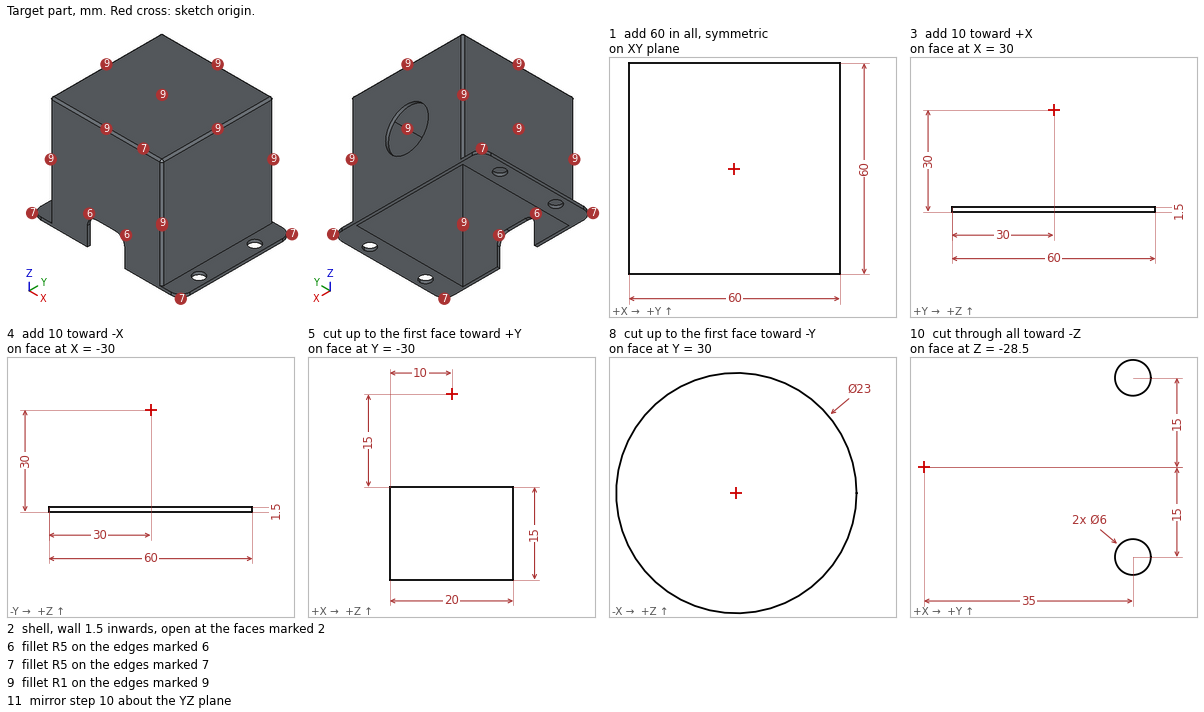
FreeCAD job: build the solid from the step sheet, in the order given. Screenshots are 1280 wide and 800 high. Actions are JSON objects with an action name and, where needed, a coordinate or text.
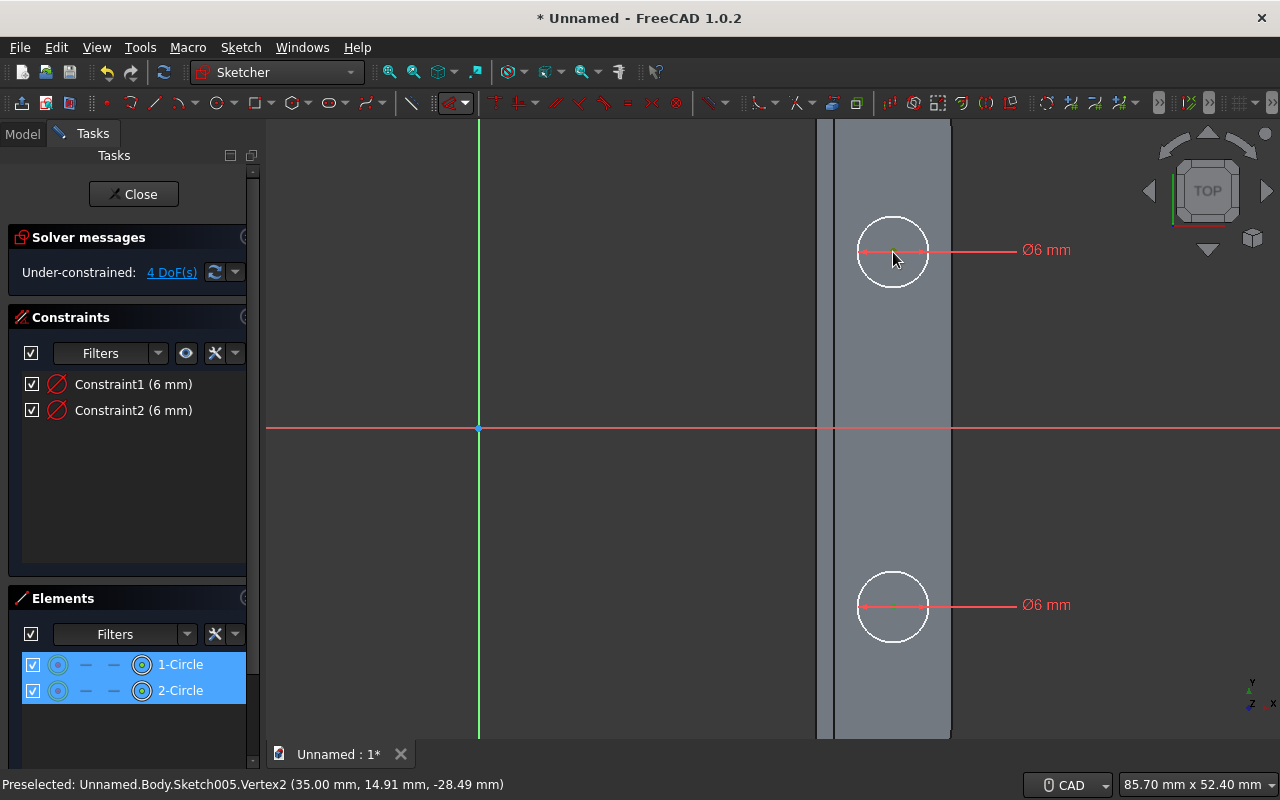
{"action": "key", "text": "v"}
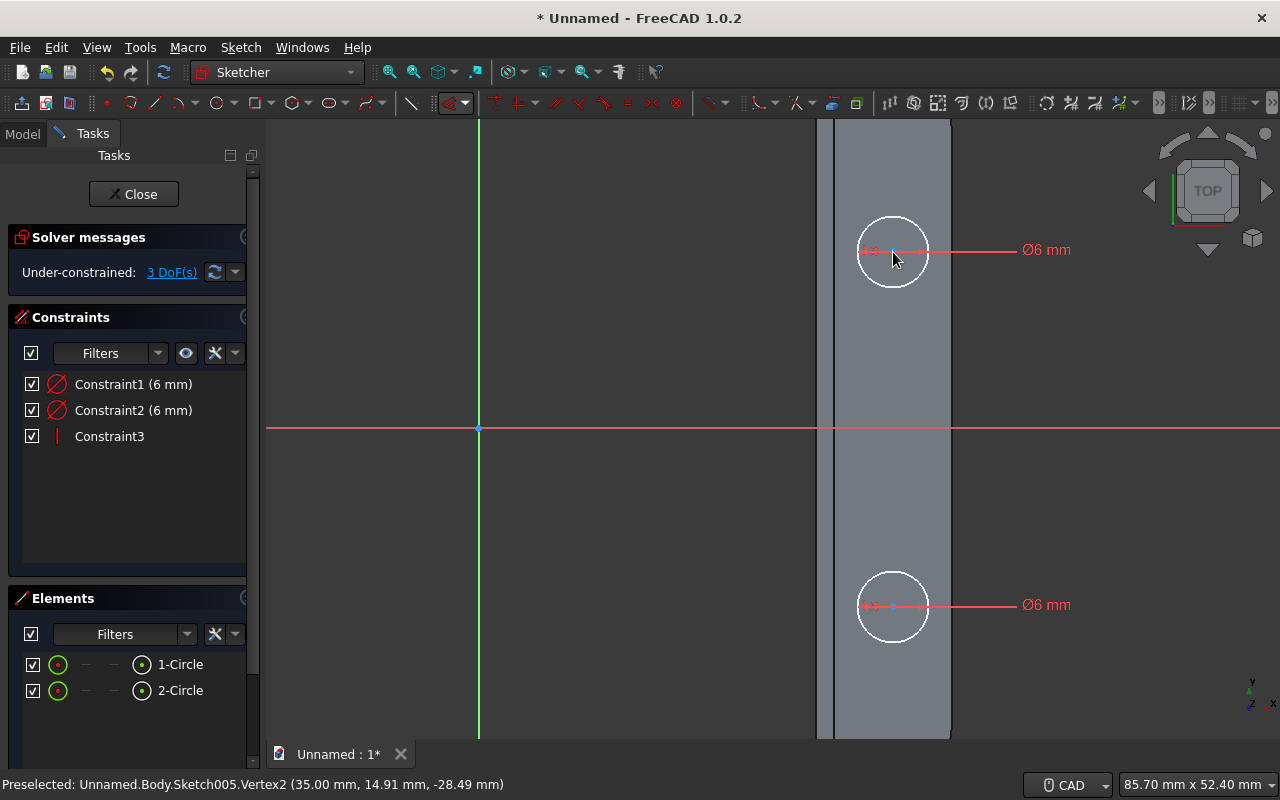
{"action": "left_click", "coordinate": [893, 607]}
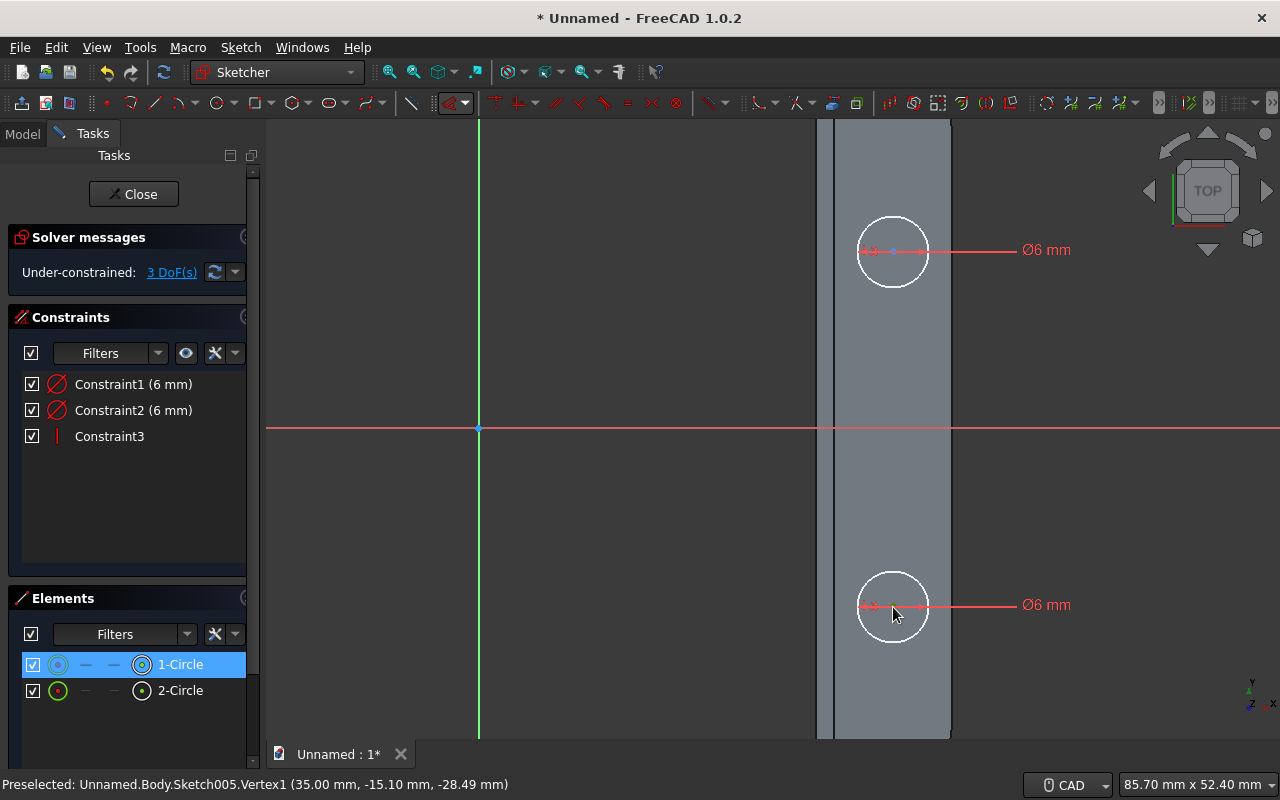
{"action": "key", "text": "l"}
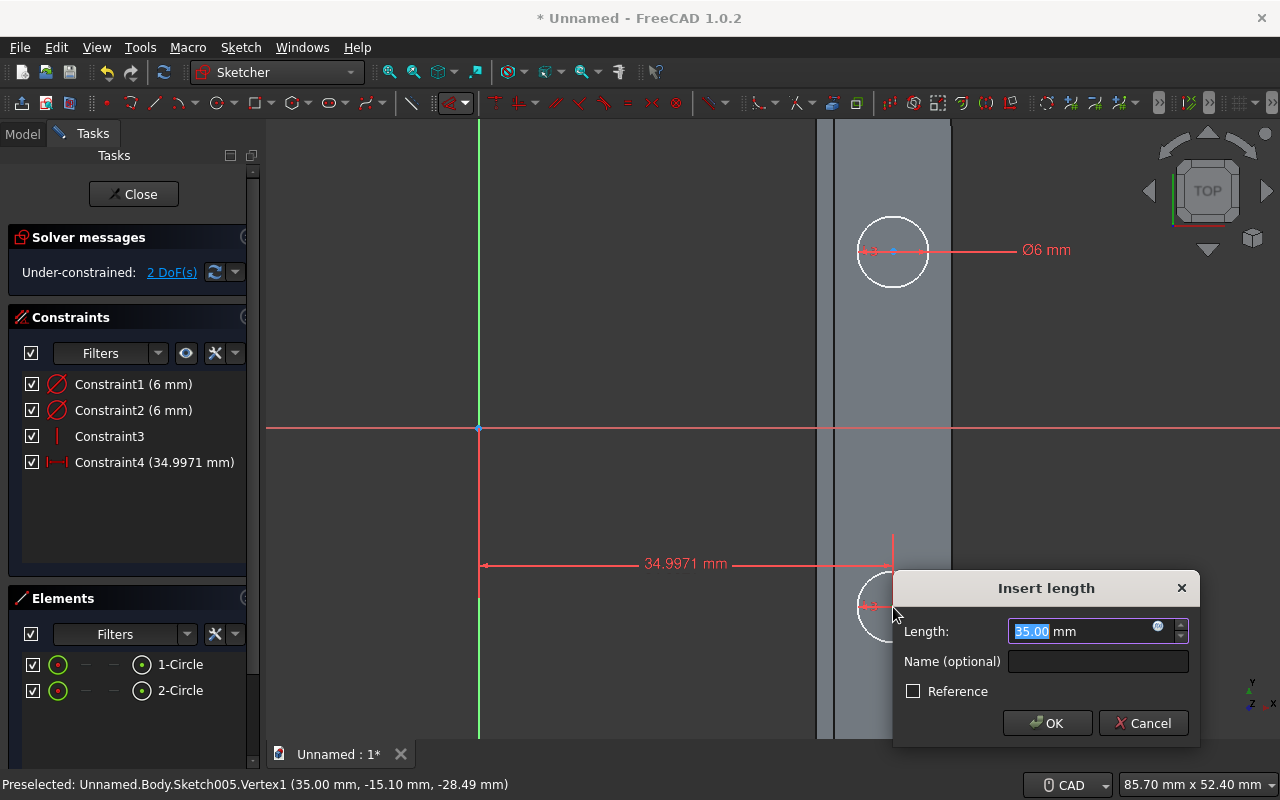
{"action": "type", "text": "35"}
{"action": "key", "text": "Return"}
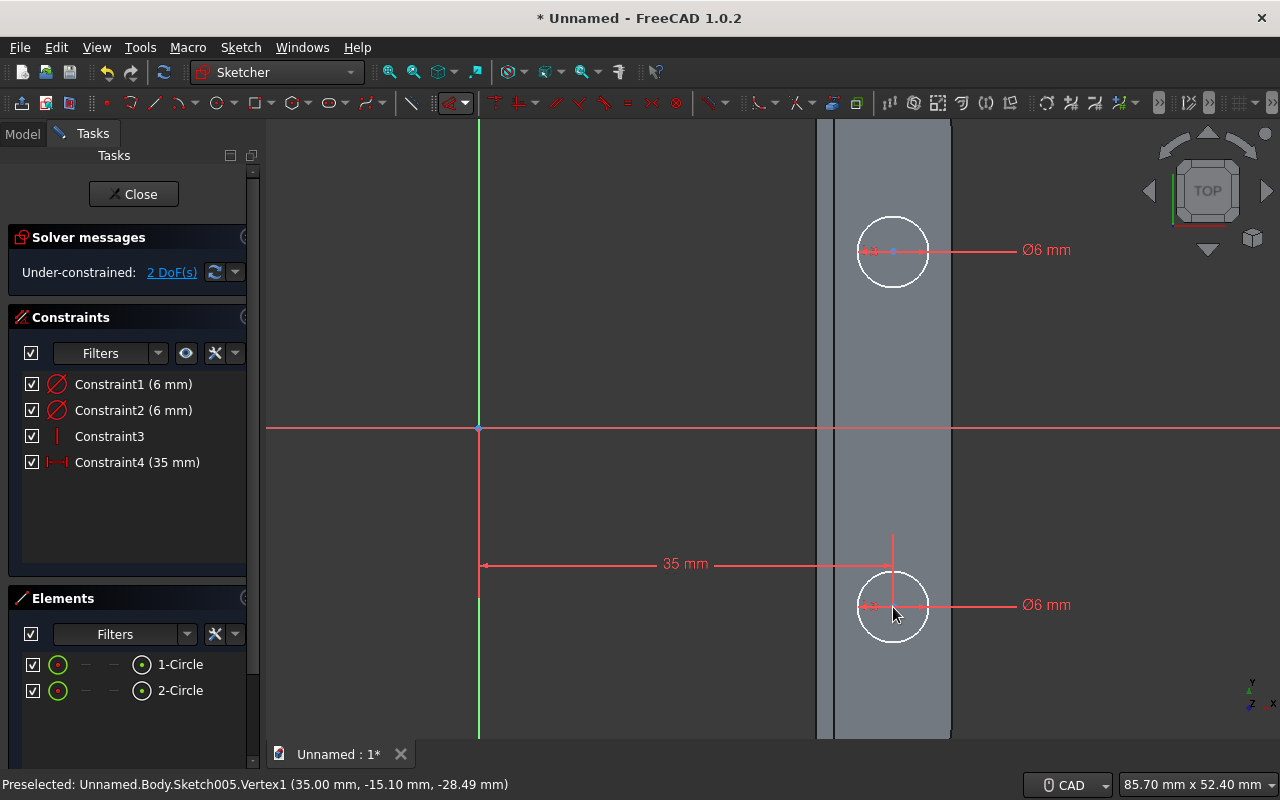
{"action": "left_click", "coordinate": [893, 607]}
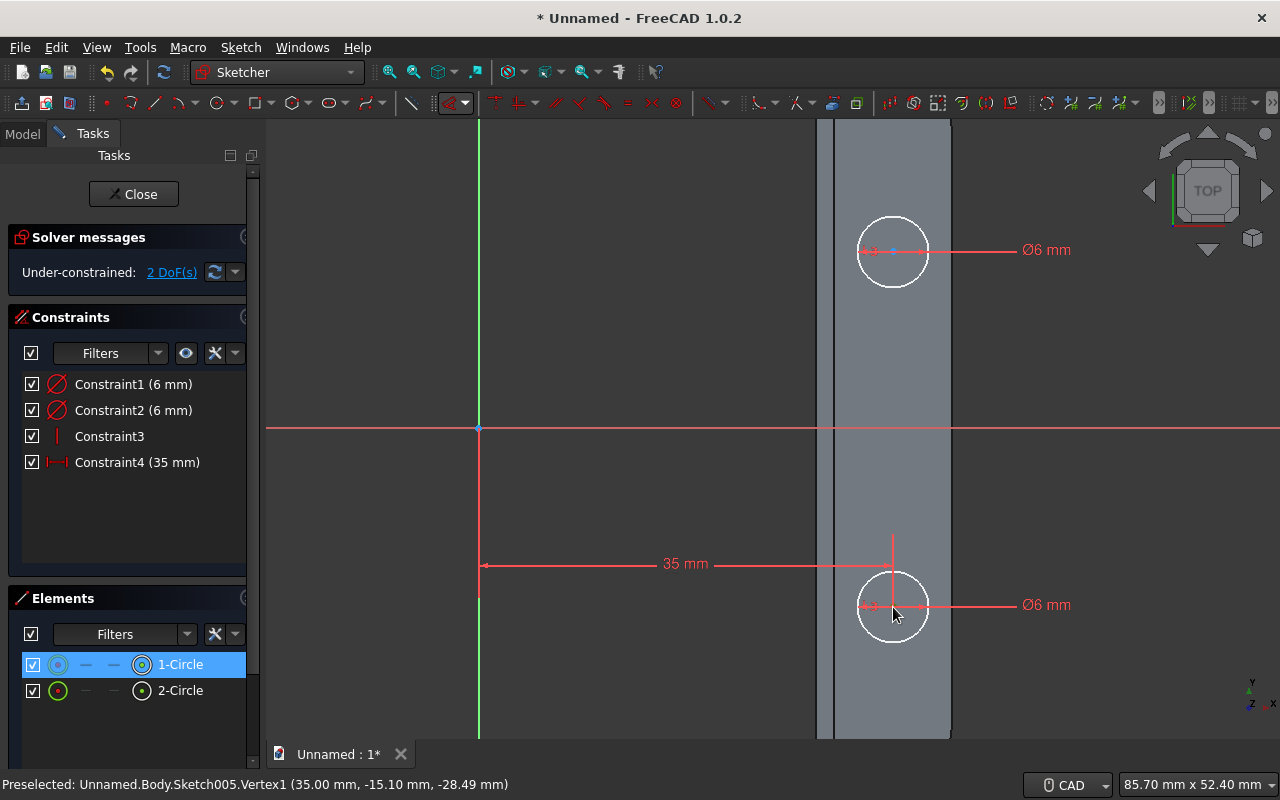
{"action": "key", "text": "i"}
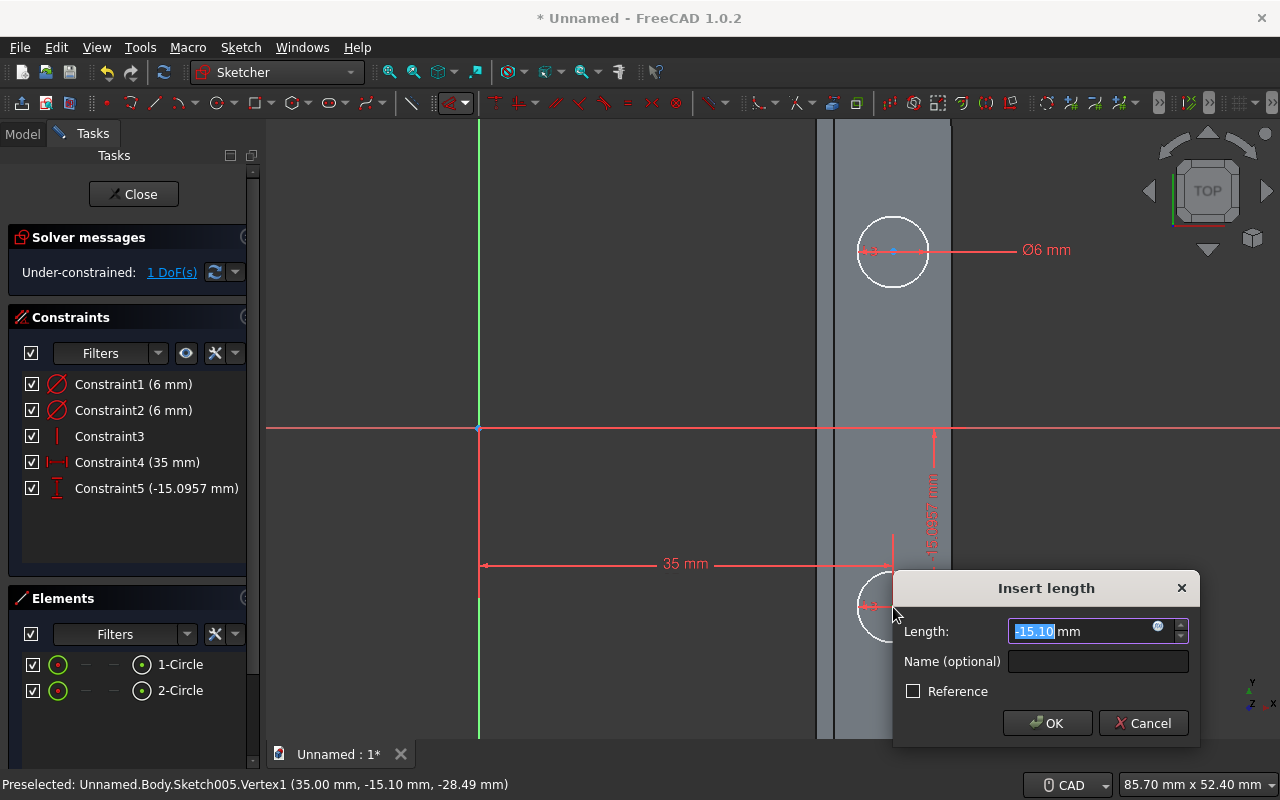
{"action": "type", "text": "-15"}
{"action": "key", "text": "Return"}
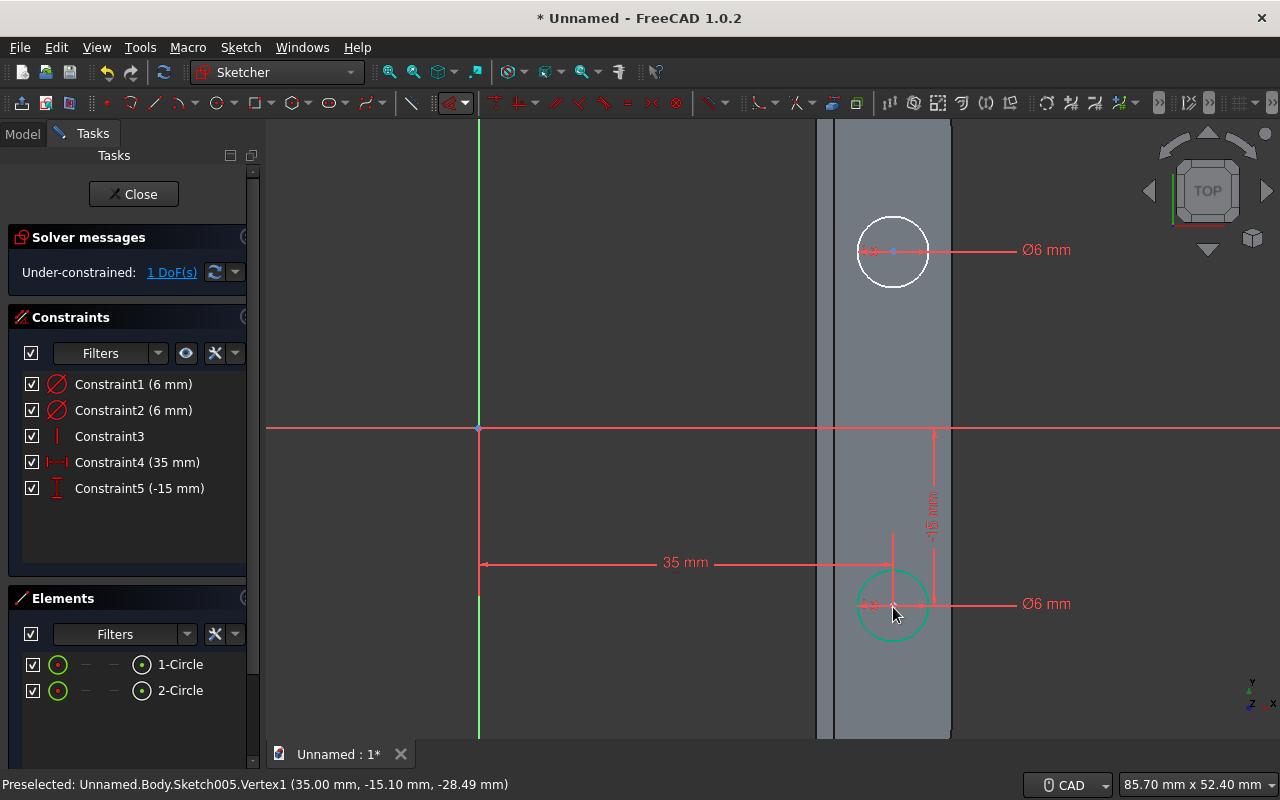
{"action": "left_click", "coordinate": [893, 252]}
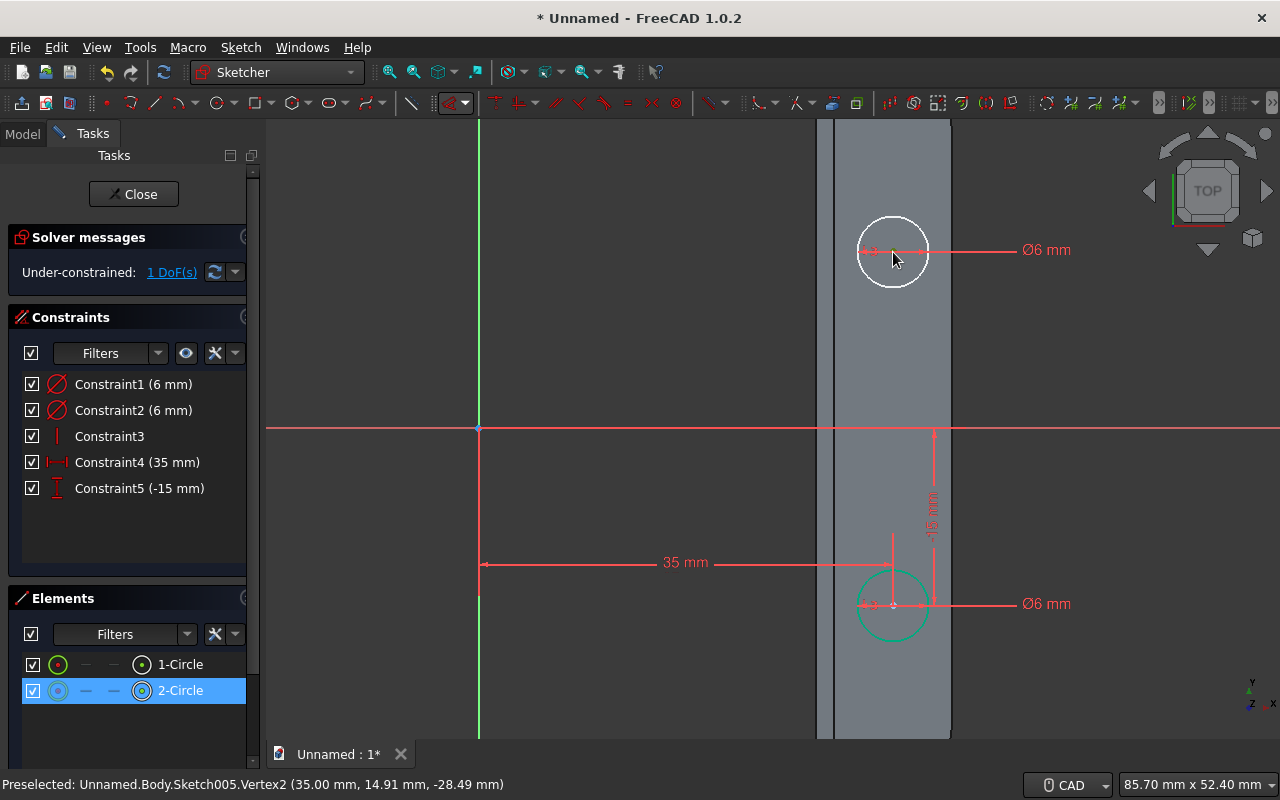
{"action": "key", "text": "i"}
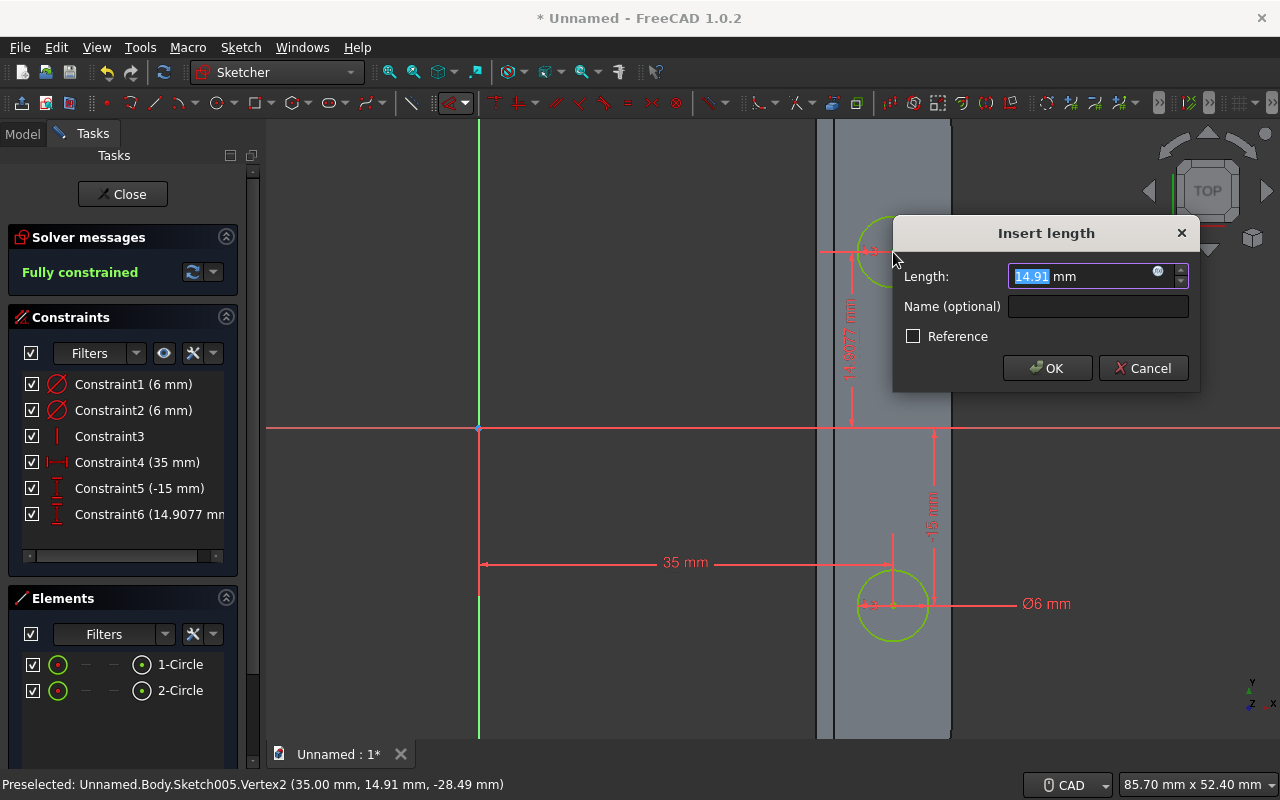
{"action": "type", "text": "15"}
{"action": "key", "text": "Return"}